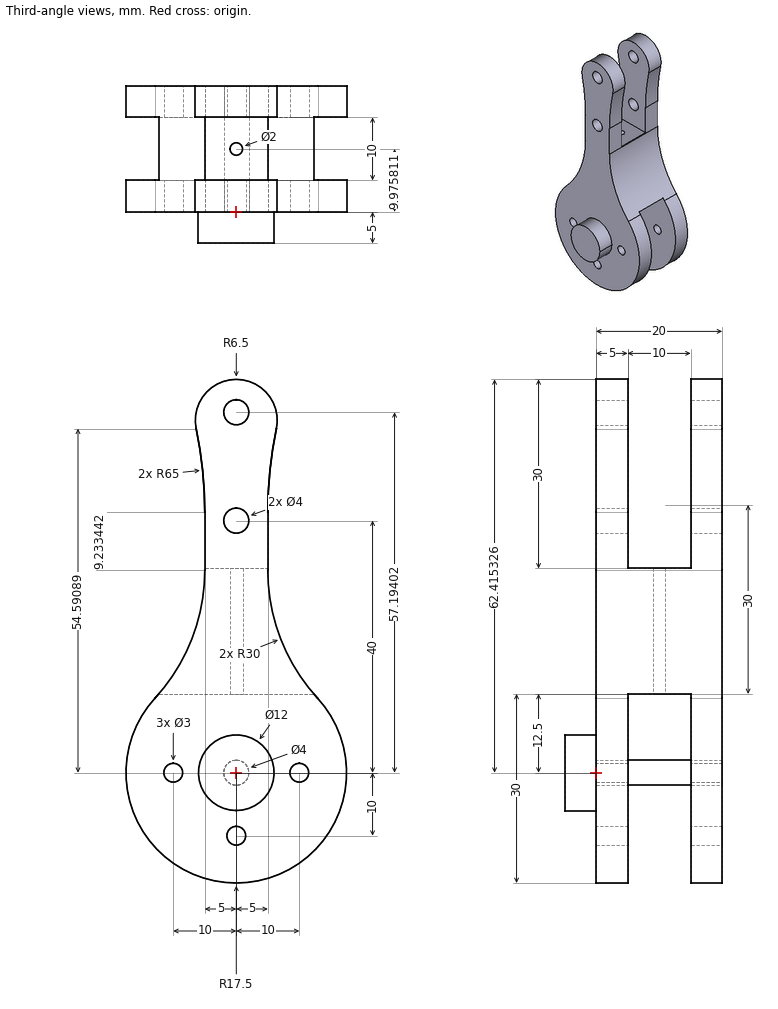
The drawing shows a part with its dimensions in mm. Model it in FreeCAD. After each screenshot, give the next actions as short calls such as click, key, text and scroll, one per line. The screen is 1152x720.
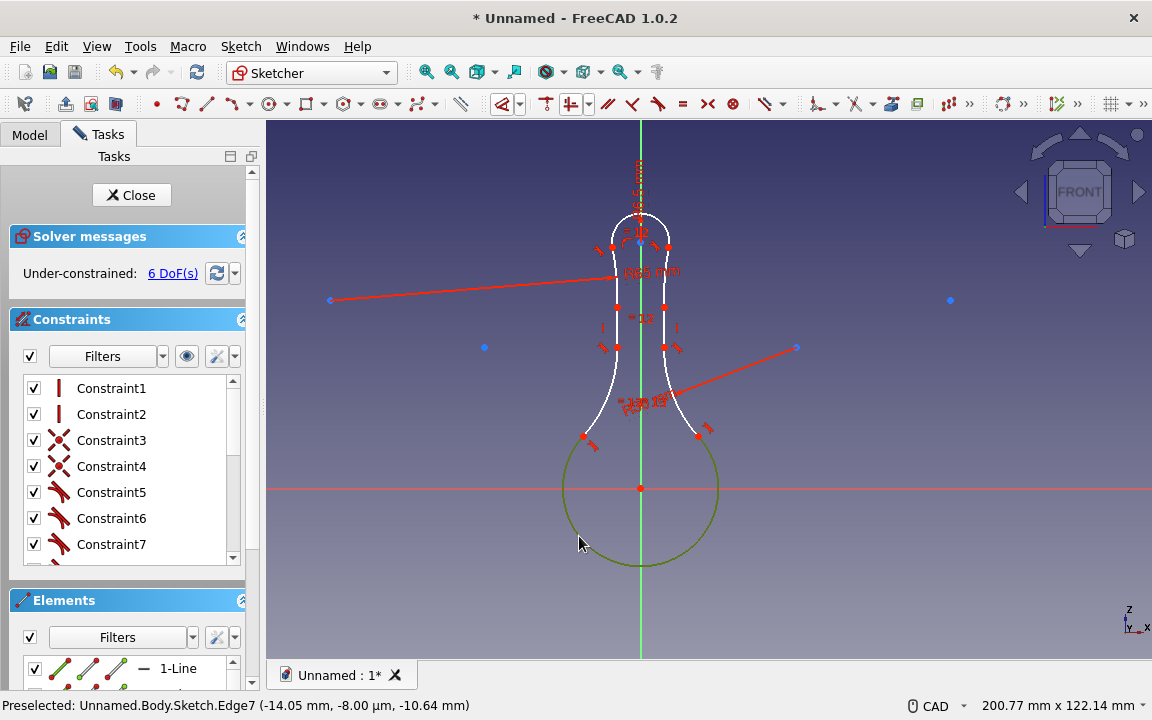
click(520, 104)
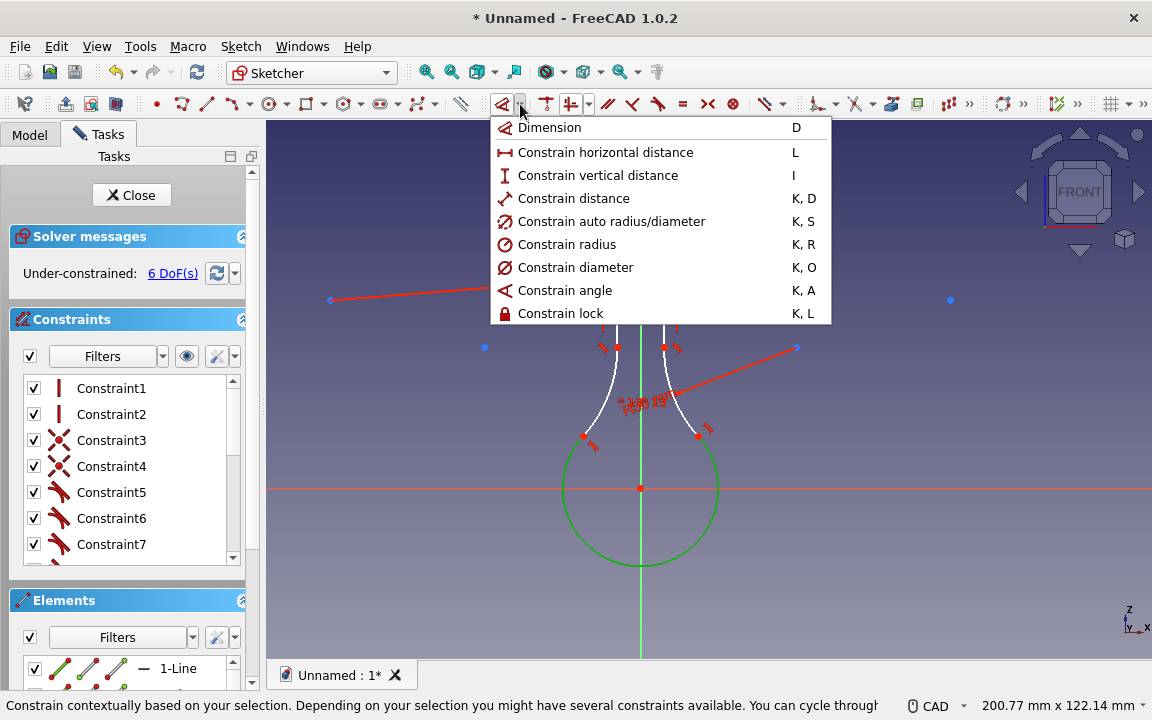
click(661, 244)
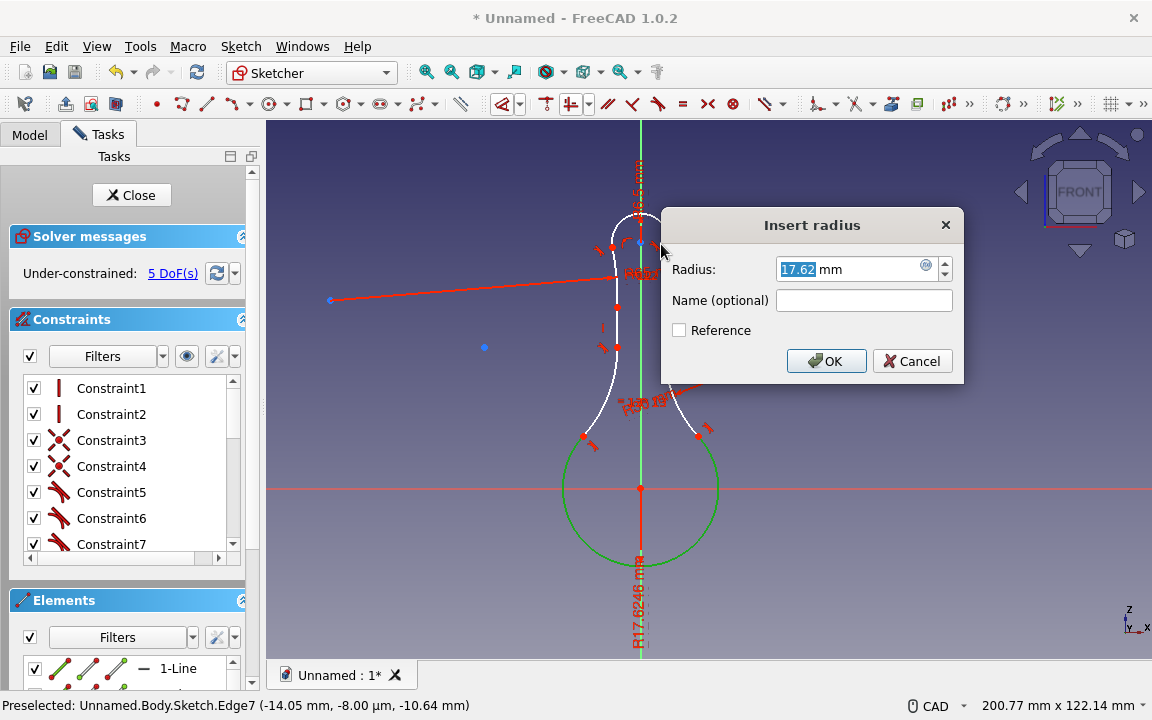
text(17.5)
key(Return)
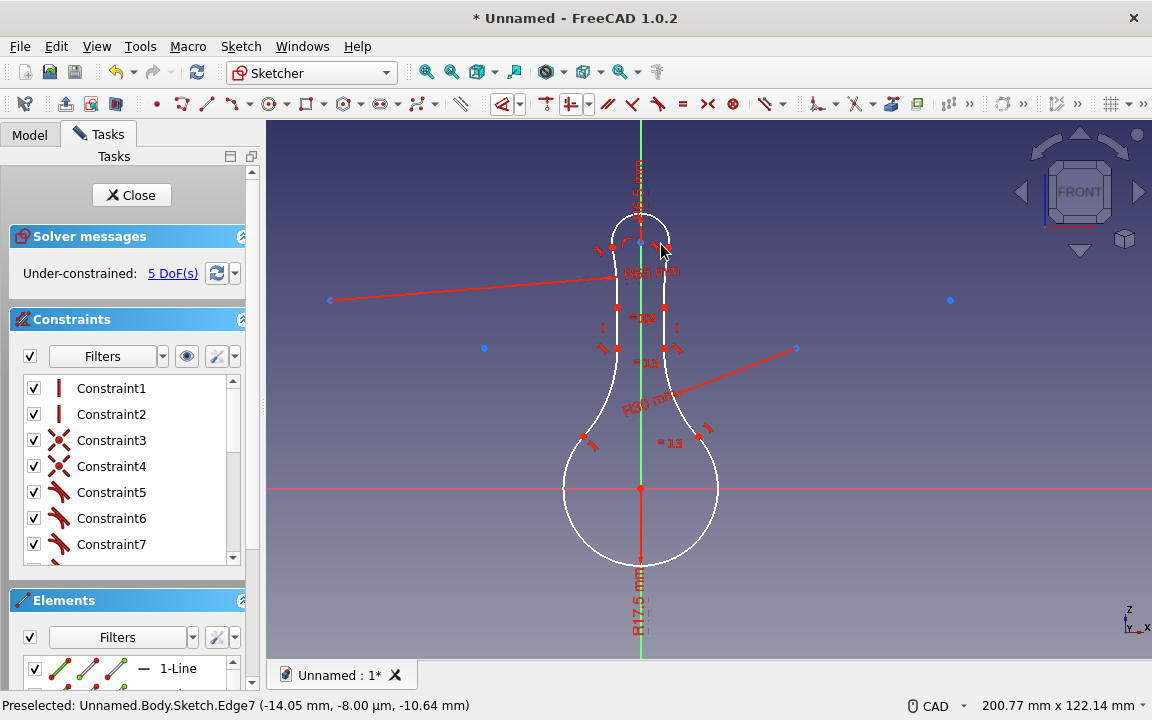
scroll(617, 348, up, 3)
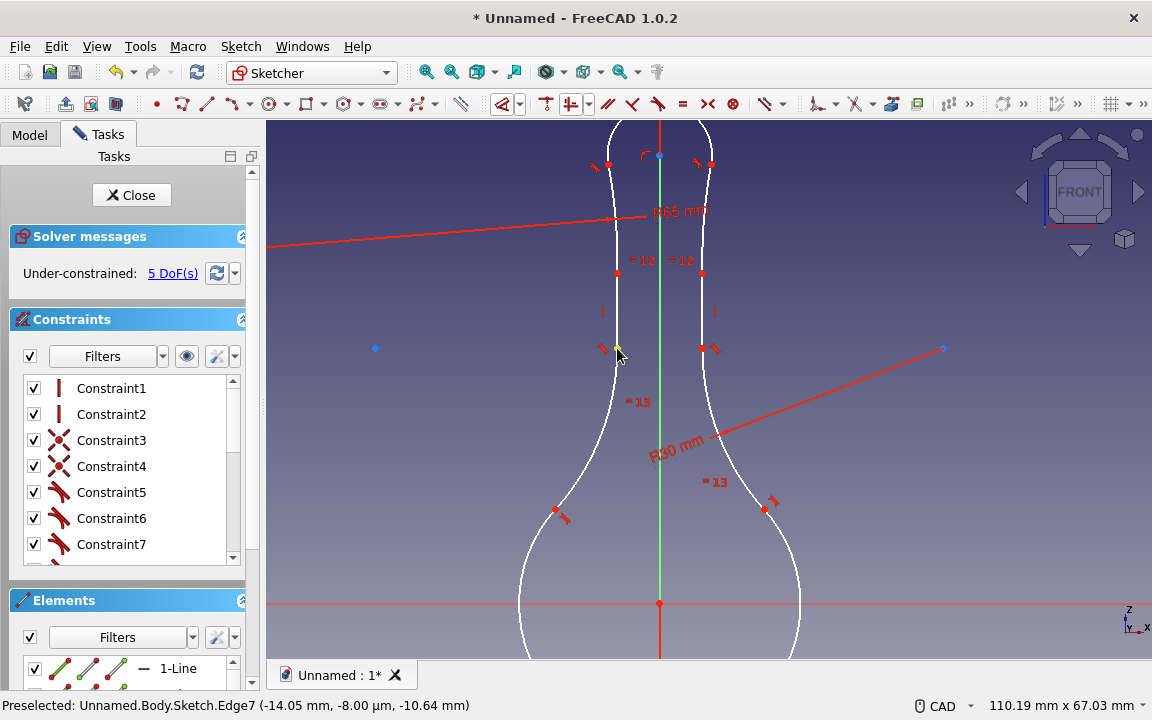
click(617, 348)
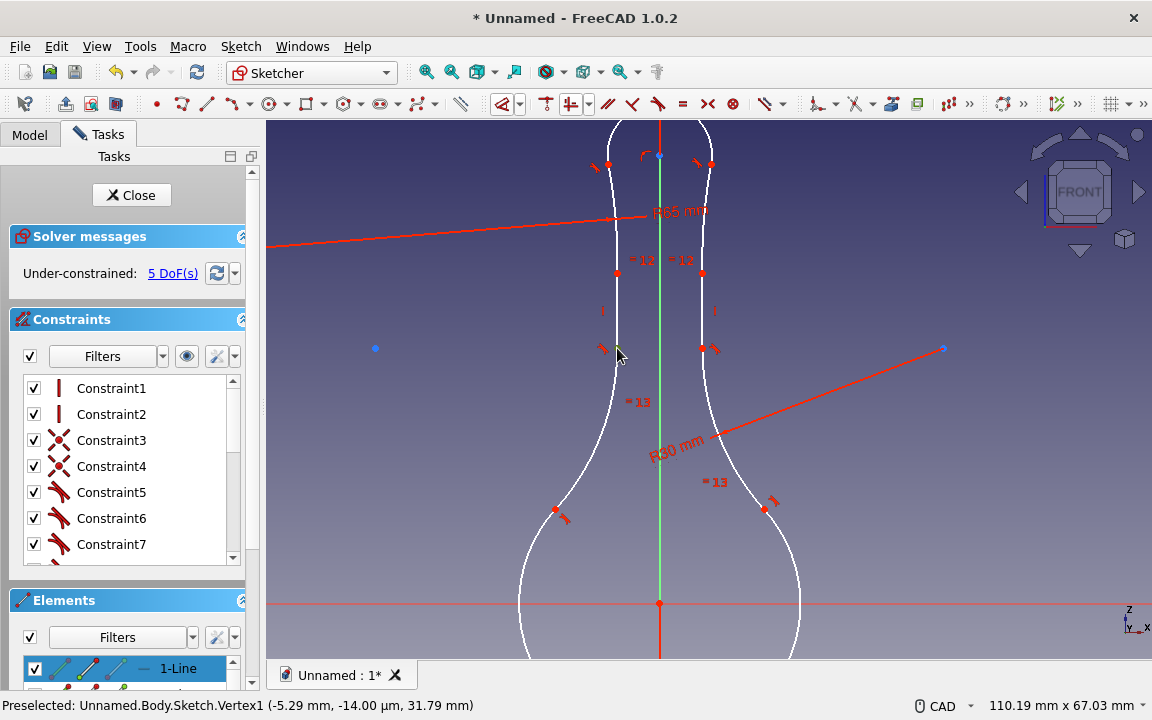
key(l)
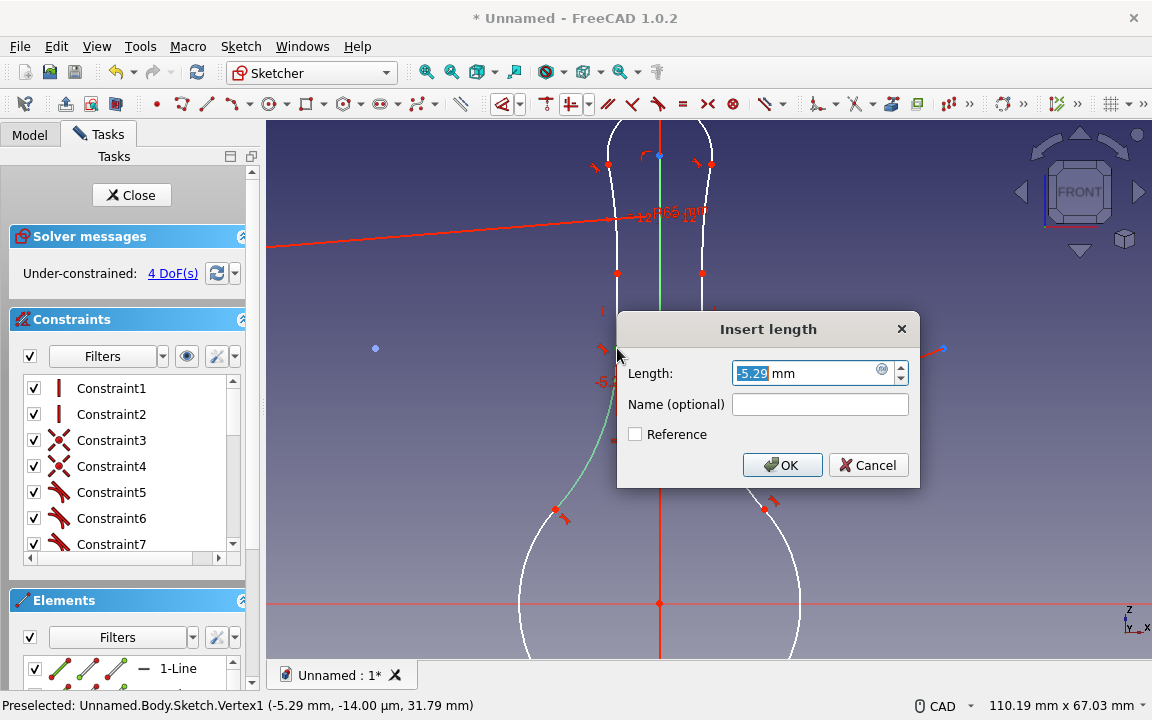
text(-5)
key(Return)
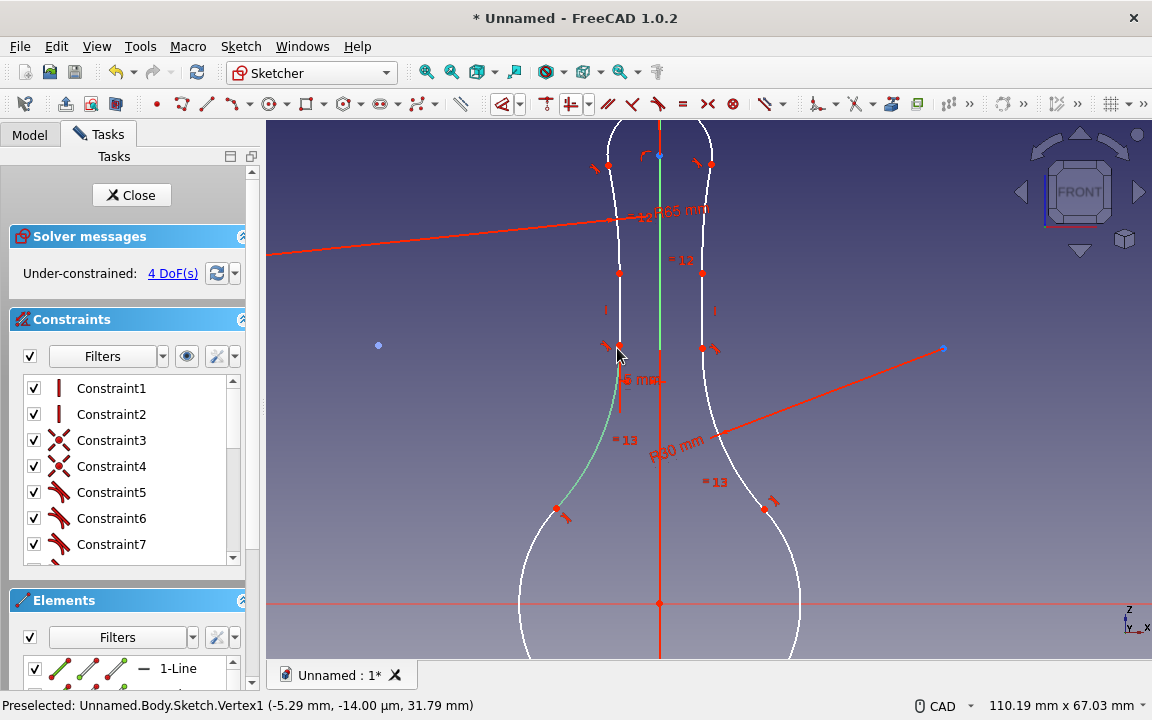
click(702, 274)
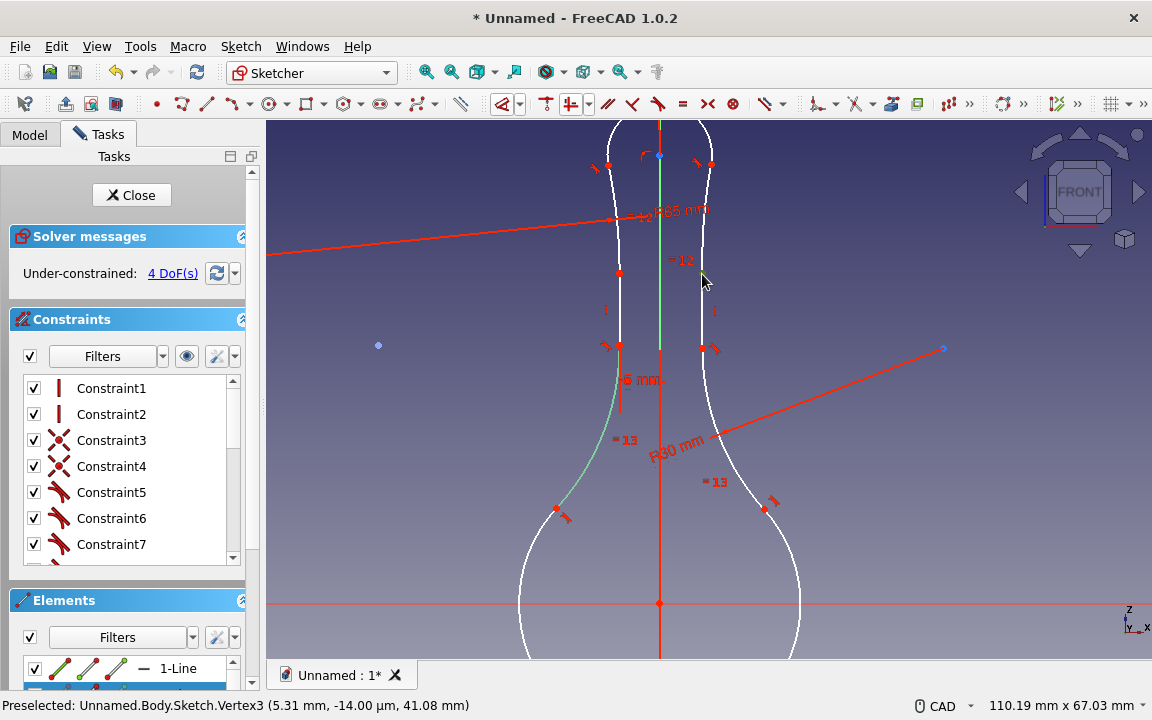
click(520, 104)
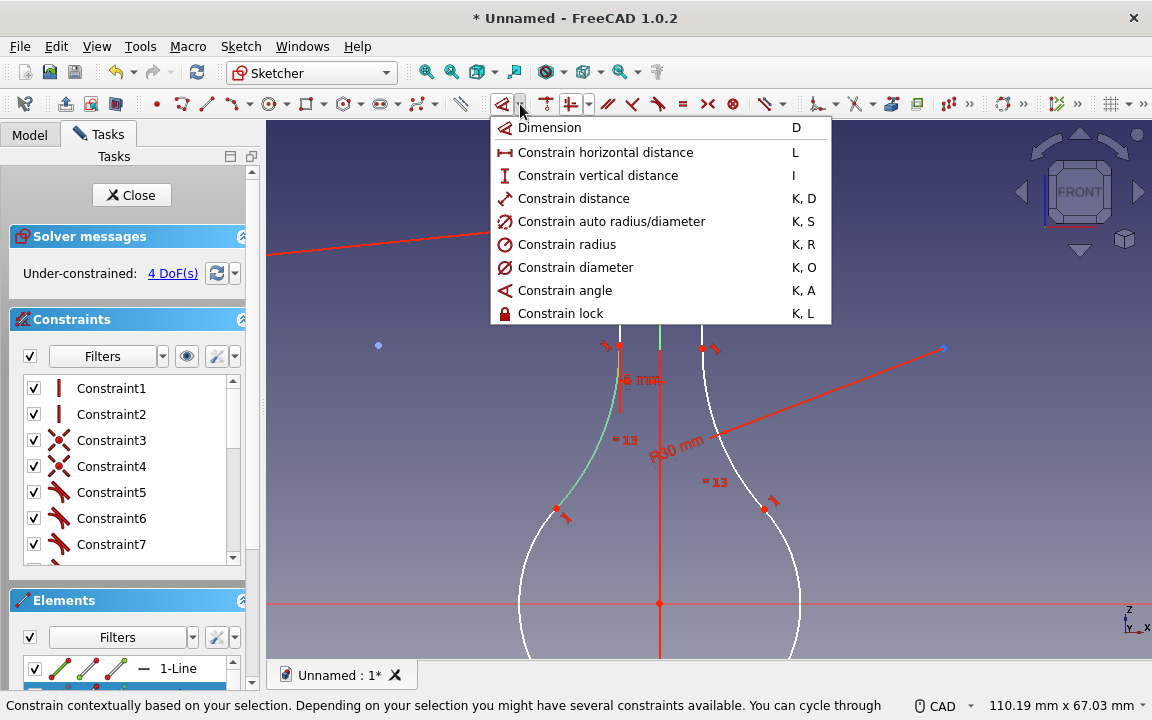
click(661, 152)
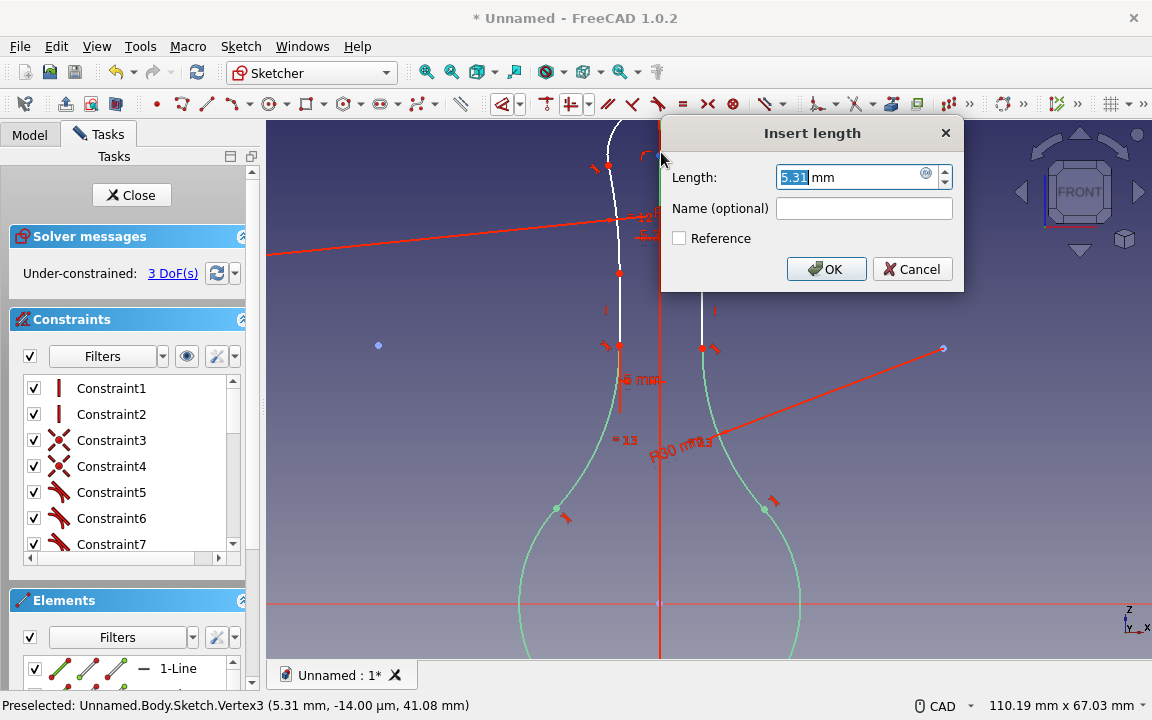
text(5)
key(Return)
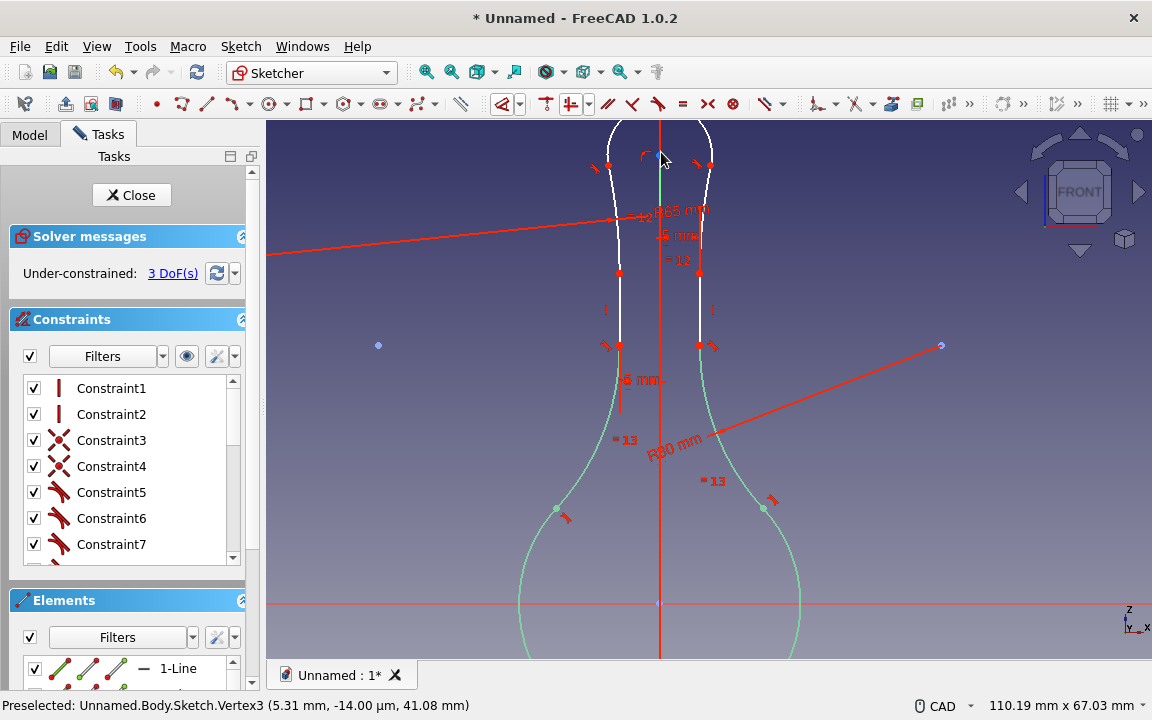
click(620, 324)